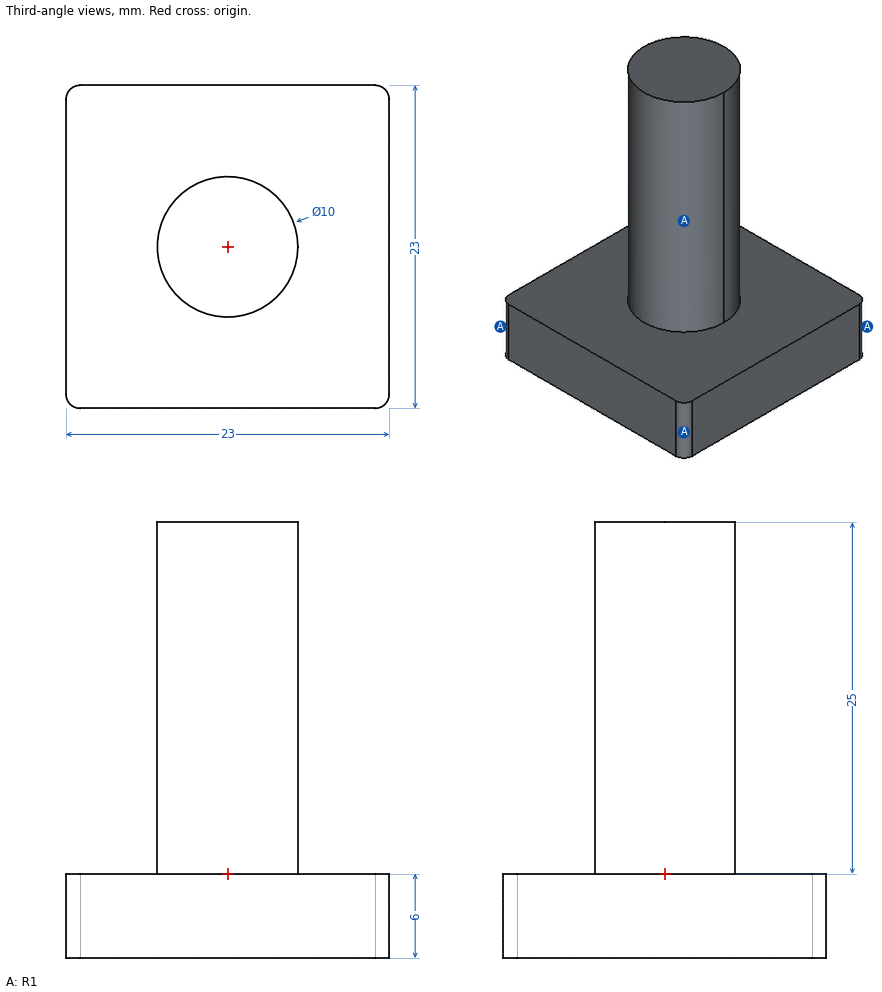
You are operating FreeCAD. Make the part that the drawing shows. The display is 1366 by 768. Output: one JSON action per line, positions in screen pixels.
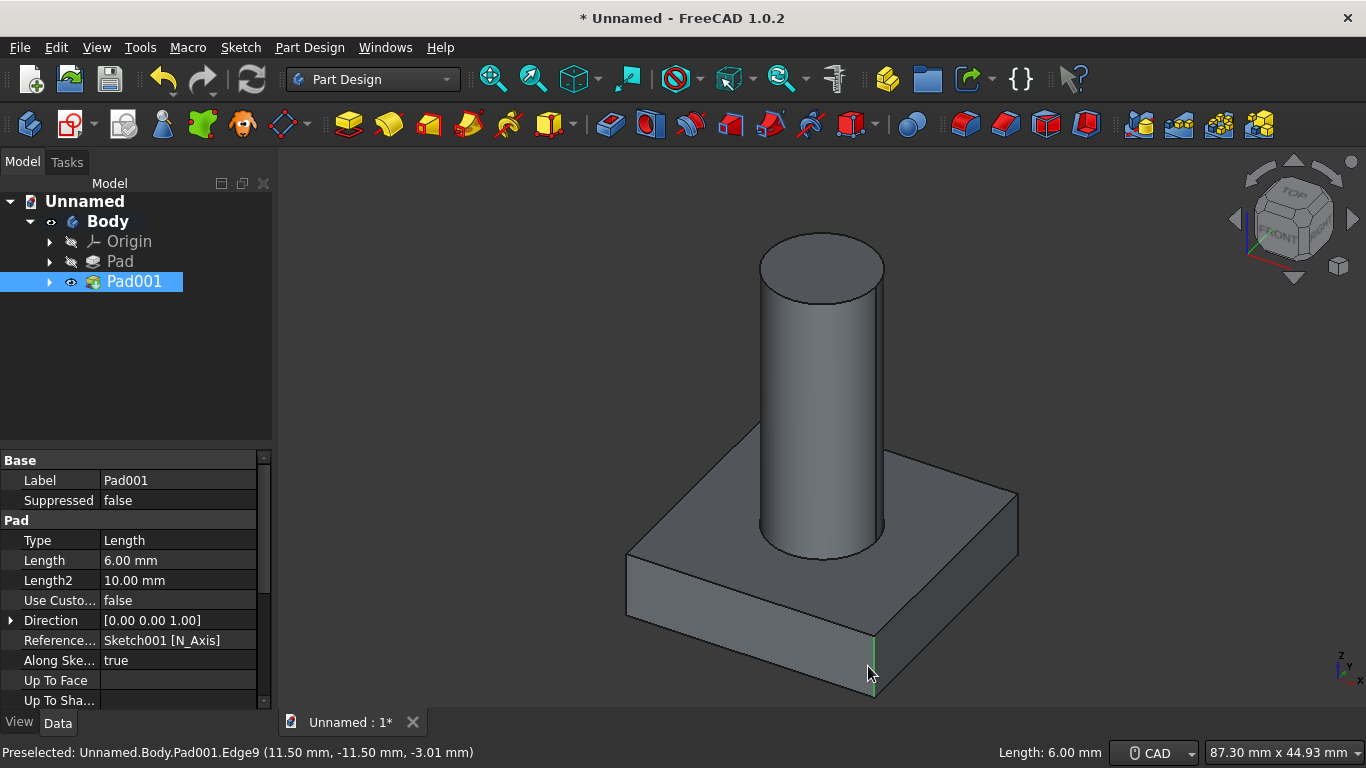
{"action": "key", "text": "0"}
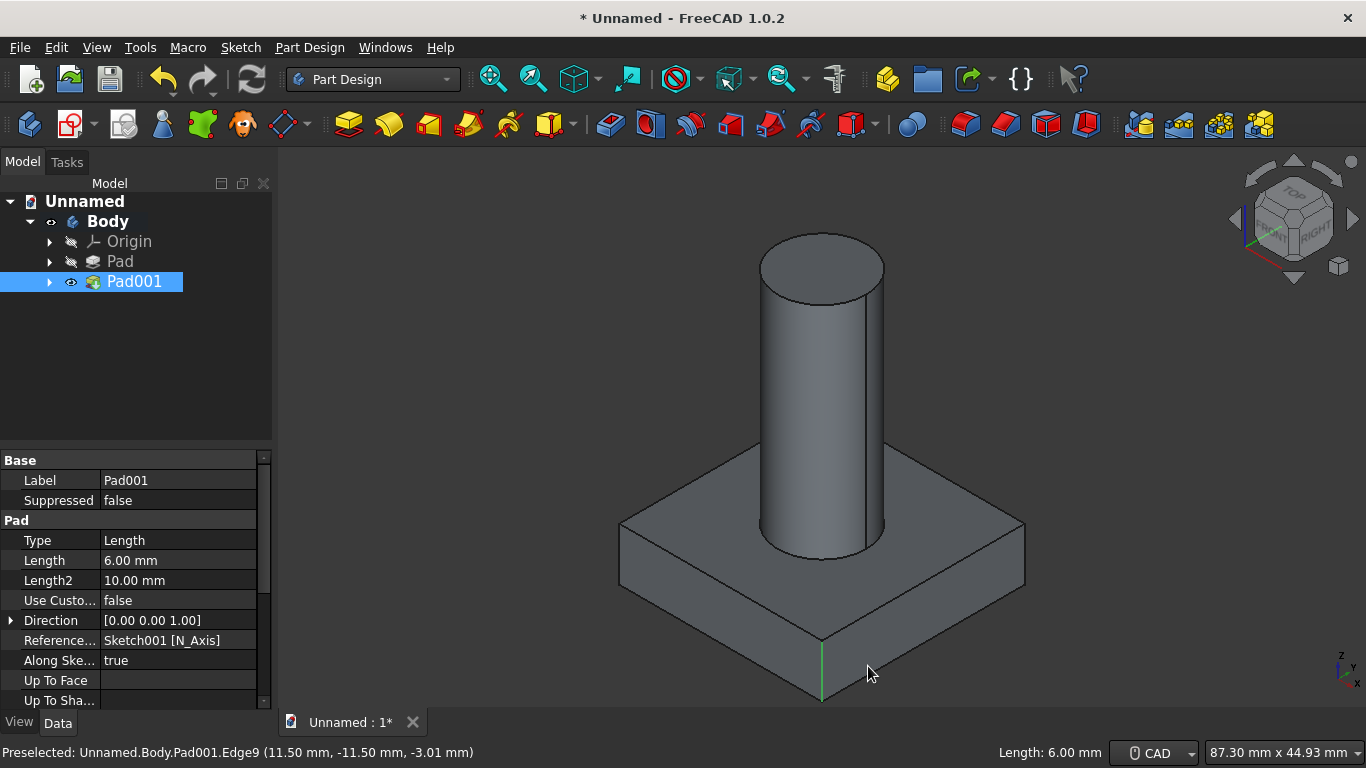
{"action": "key", "text": "2"}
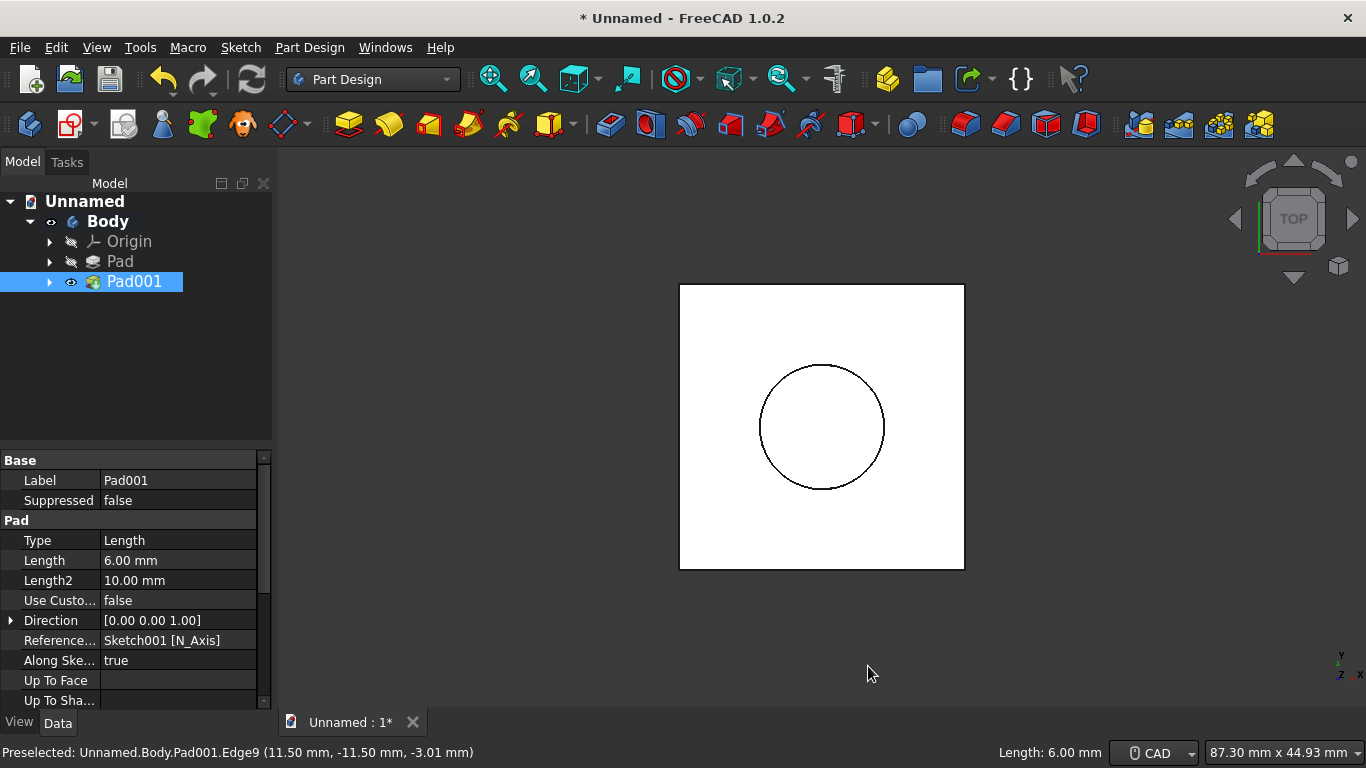
{"action": "key", "text": "1"}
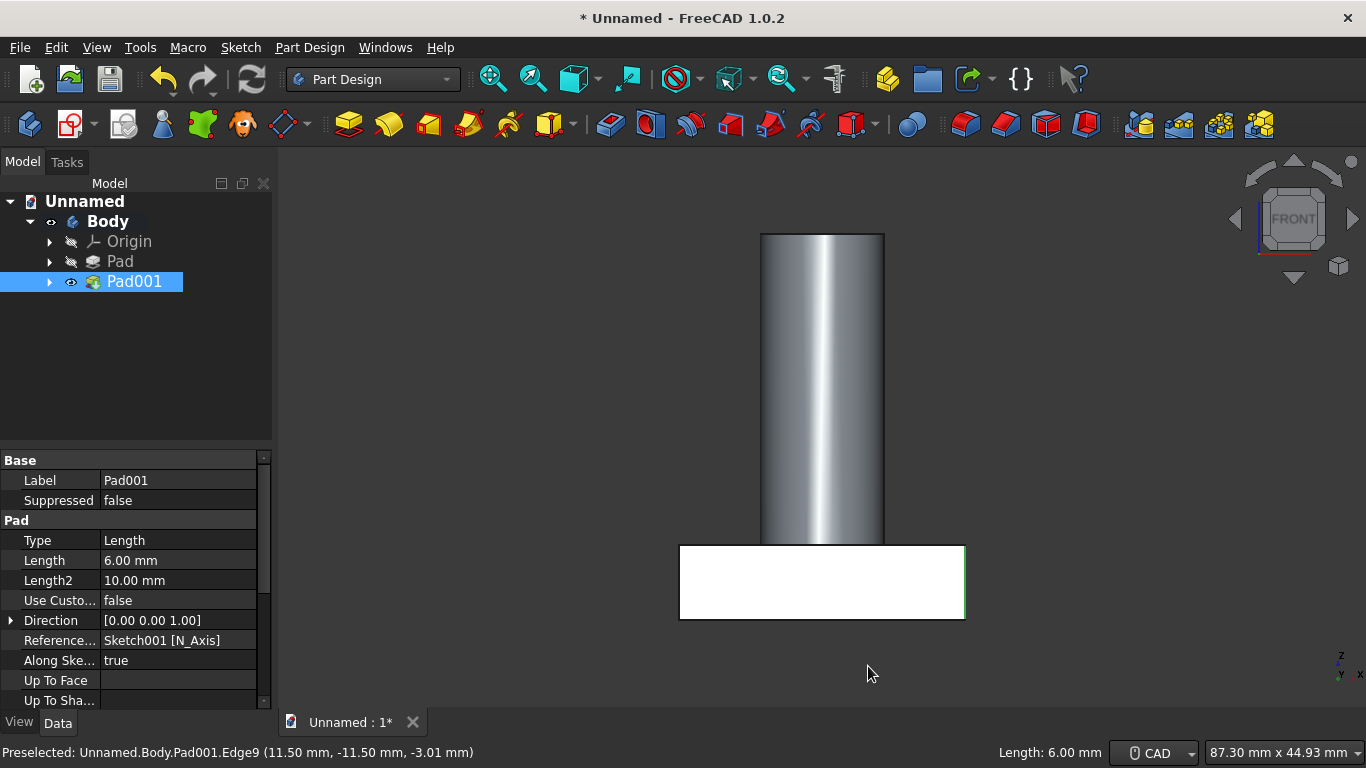
{"action": "left_click", "coordinate": [679, 582], "text": "ctrl"}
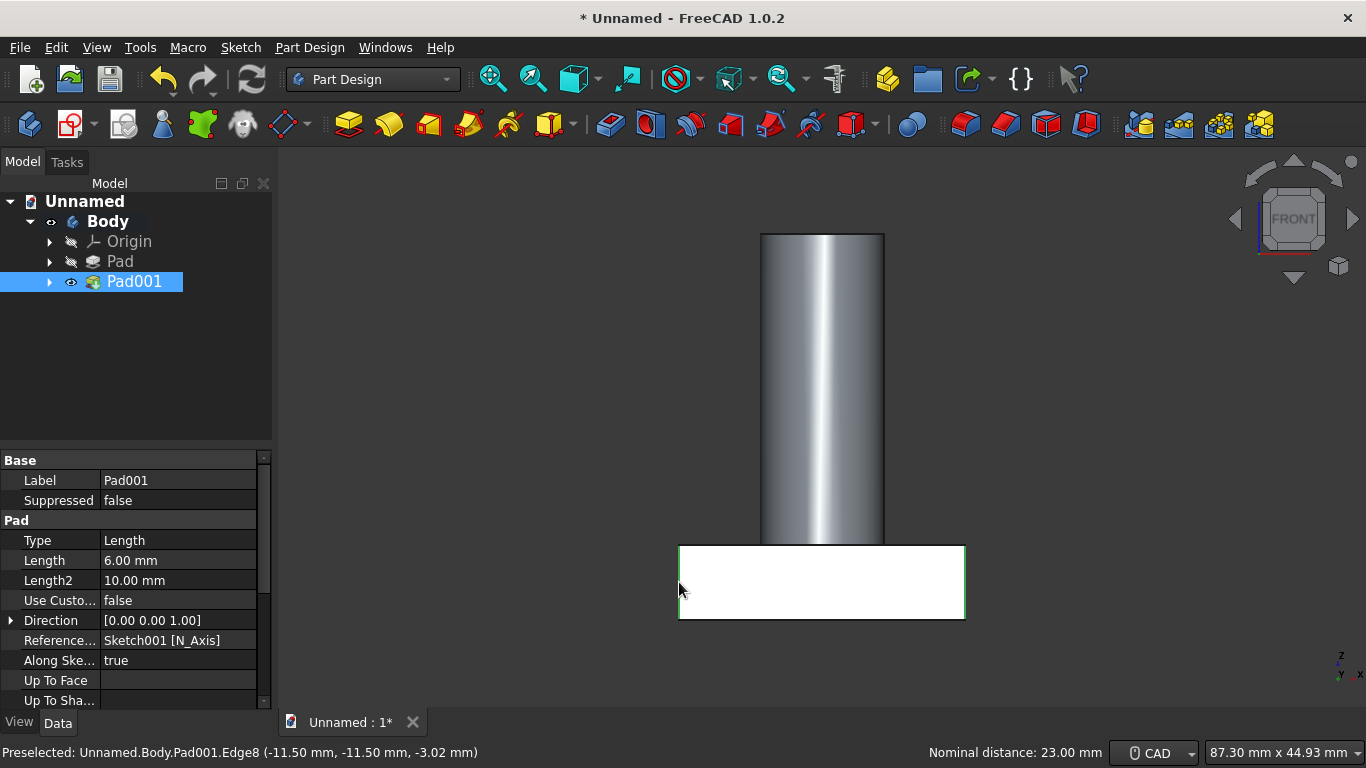
{"action": "key", "text": "3"}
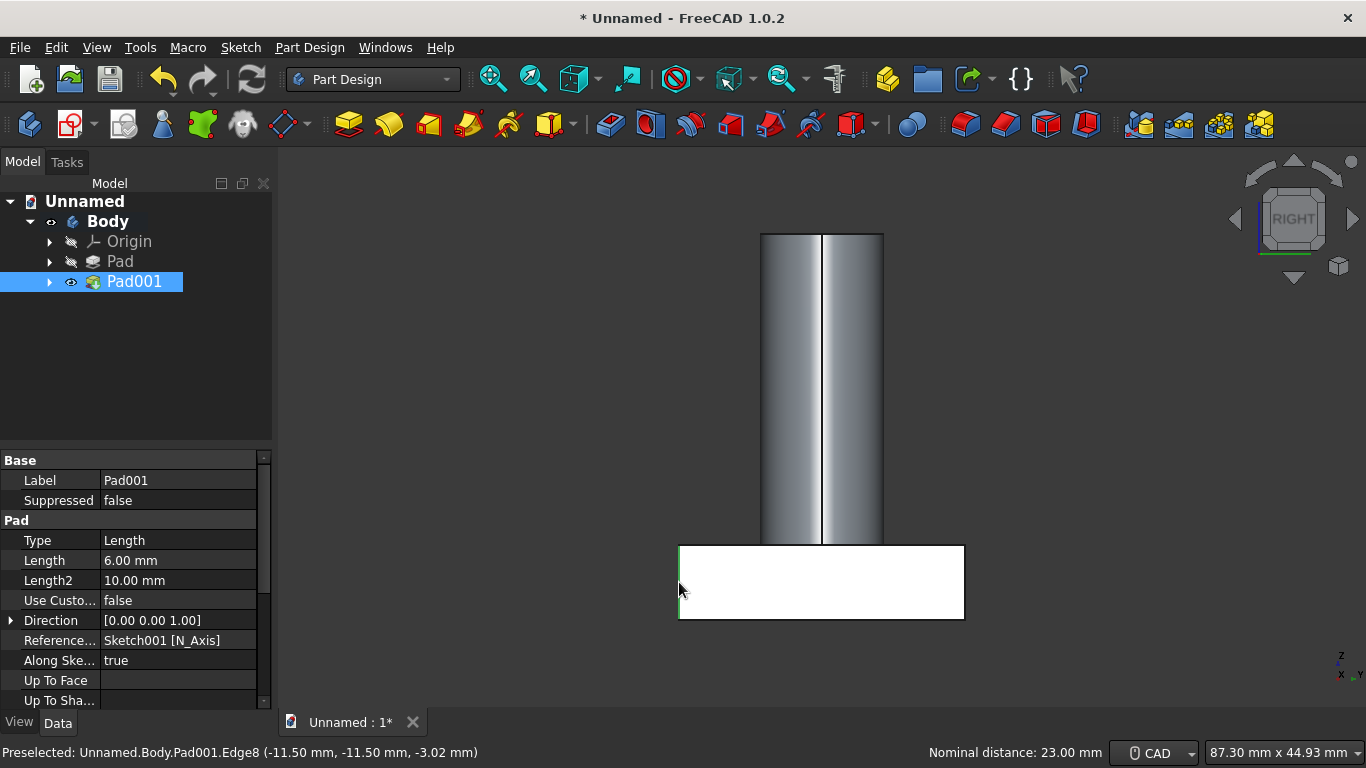
{"action": "left_click", "coordinate": [965, 582], "text": "ctrl"}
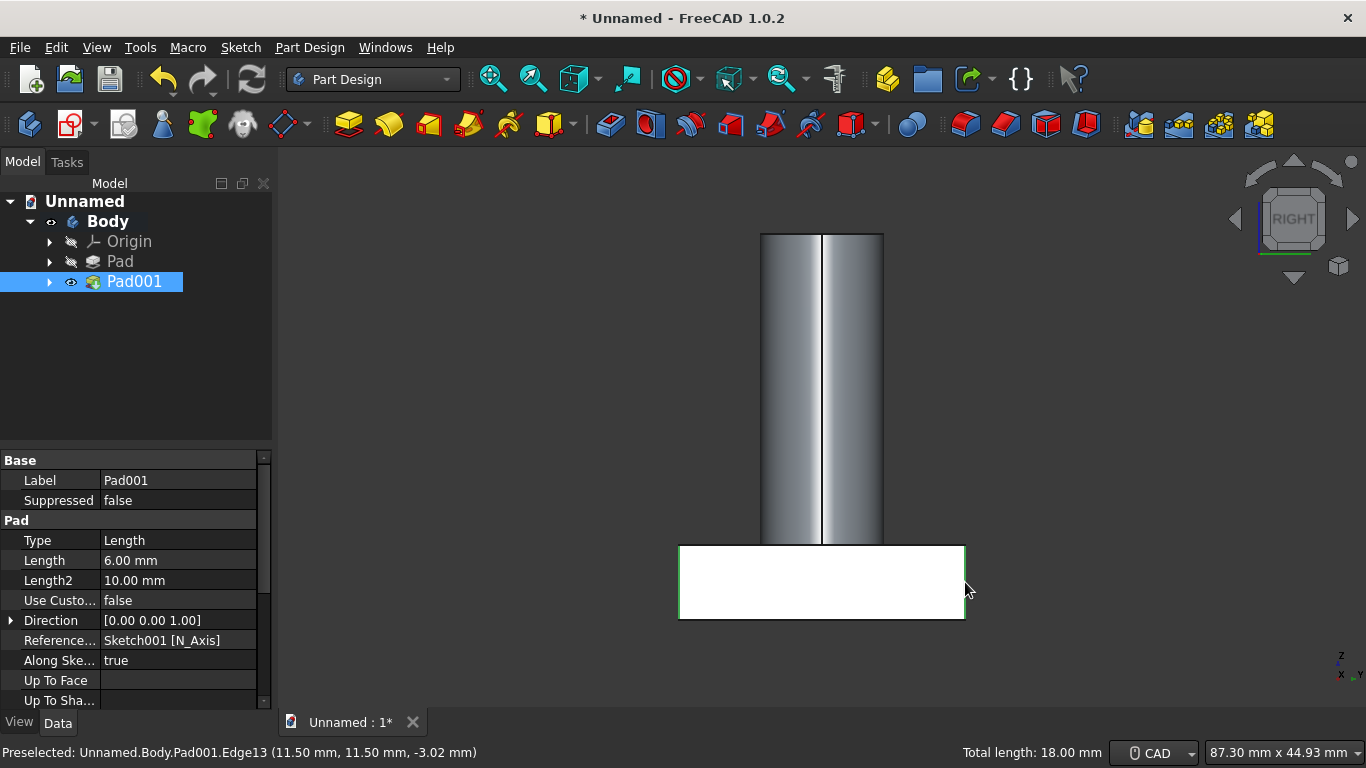
{"action": "key", "text": "5"}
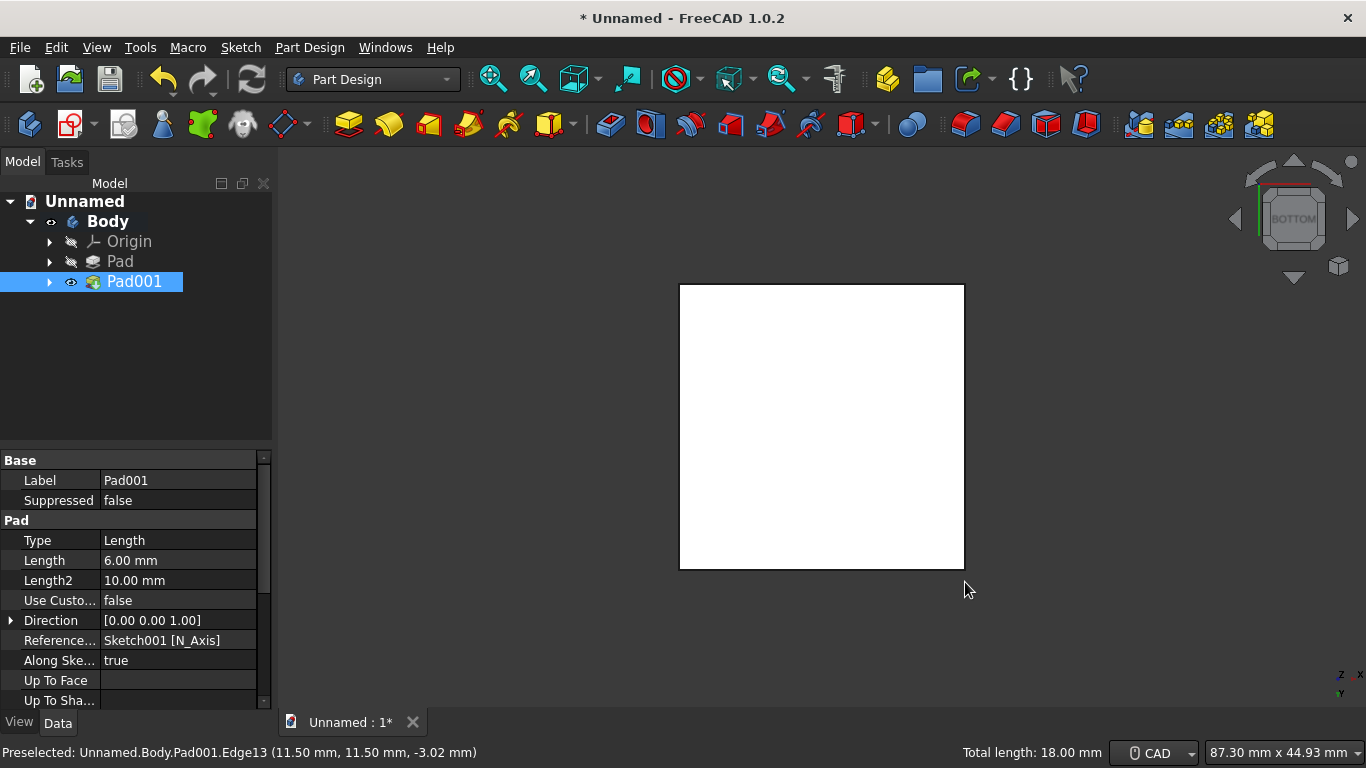
{"action": "key", "text": "4"}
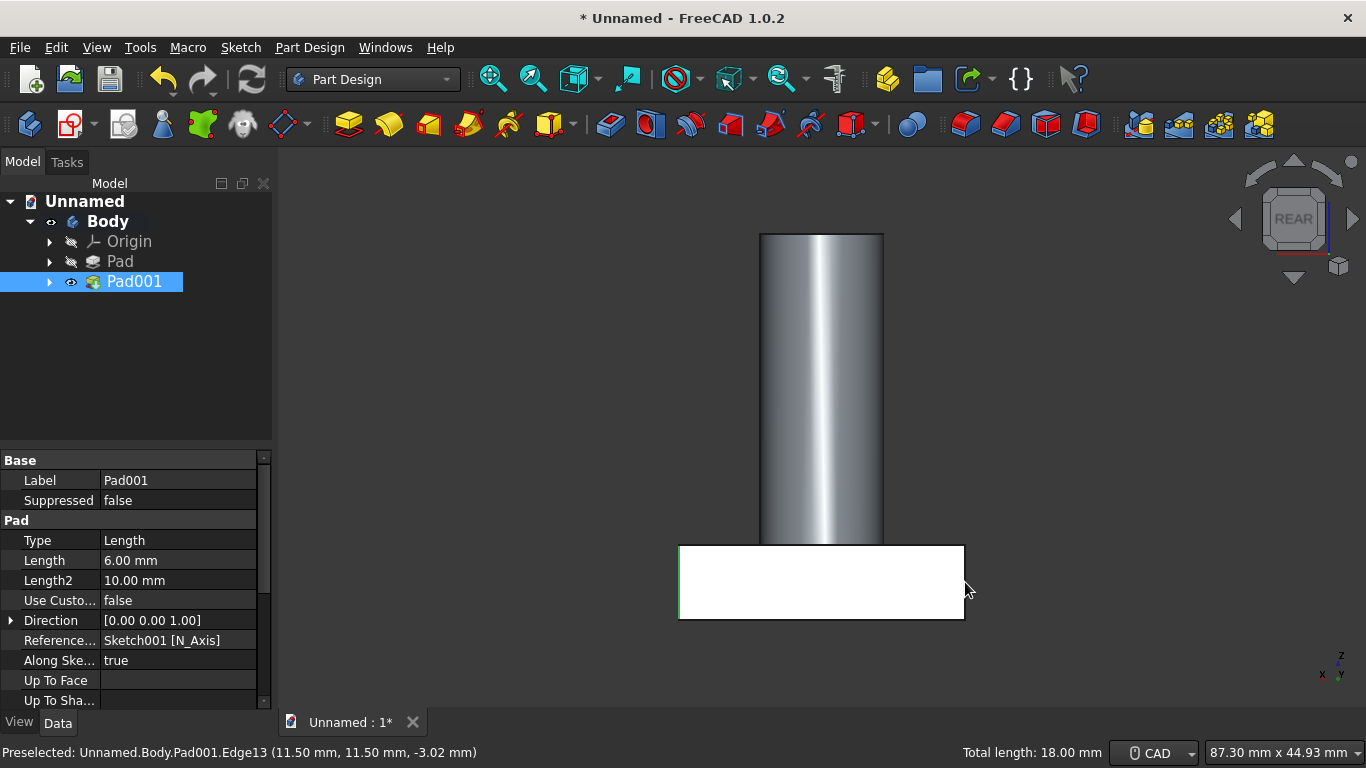
{"action": "left_click", "coordinate": [965, 582], "text": "ctrl"}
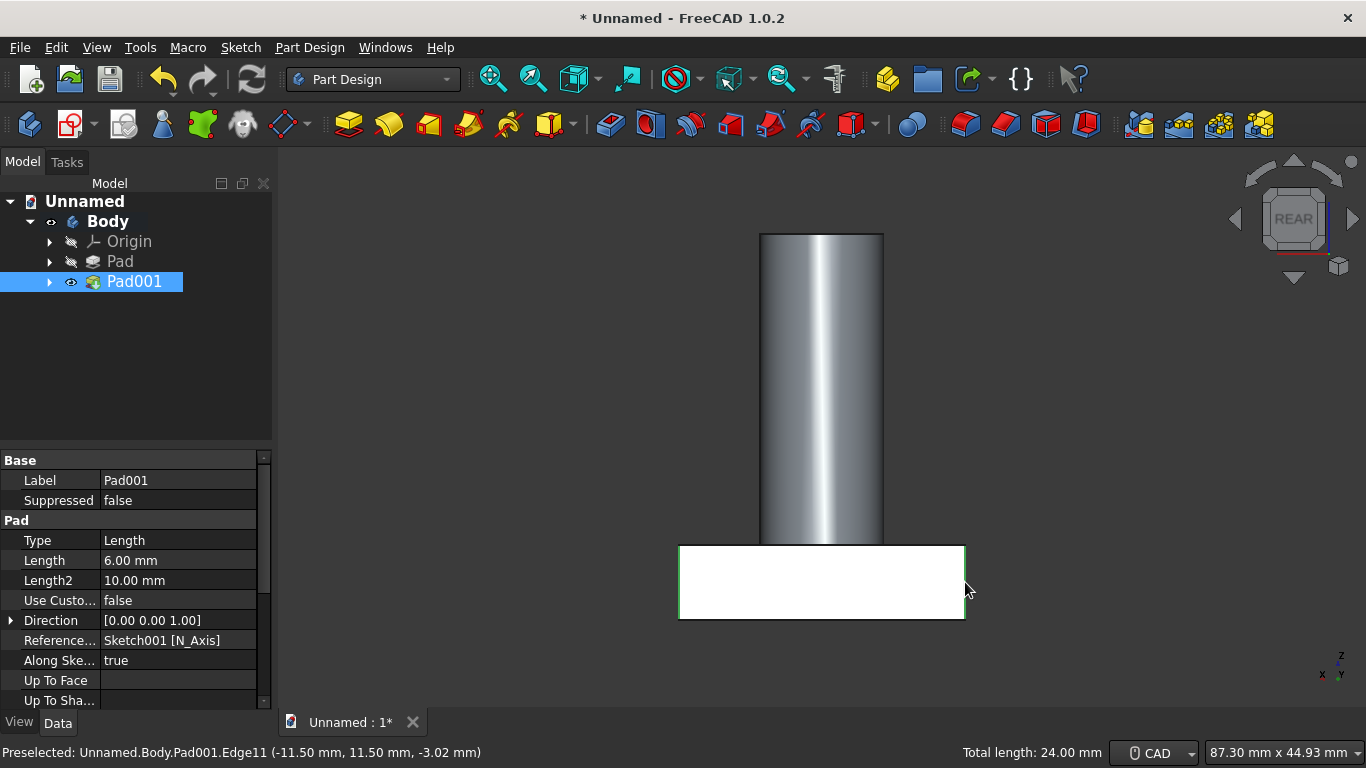
{"action": "left_click", "coordinate": [966, 124]}